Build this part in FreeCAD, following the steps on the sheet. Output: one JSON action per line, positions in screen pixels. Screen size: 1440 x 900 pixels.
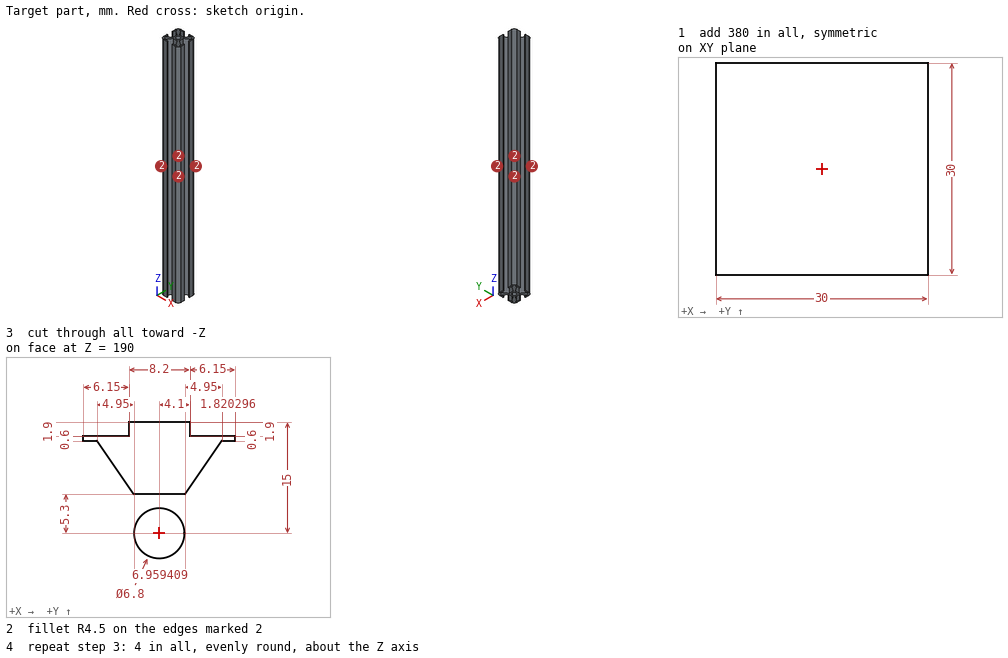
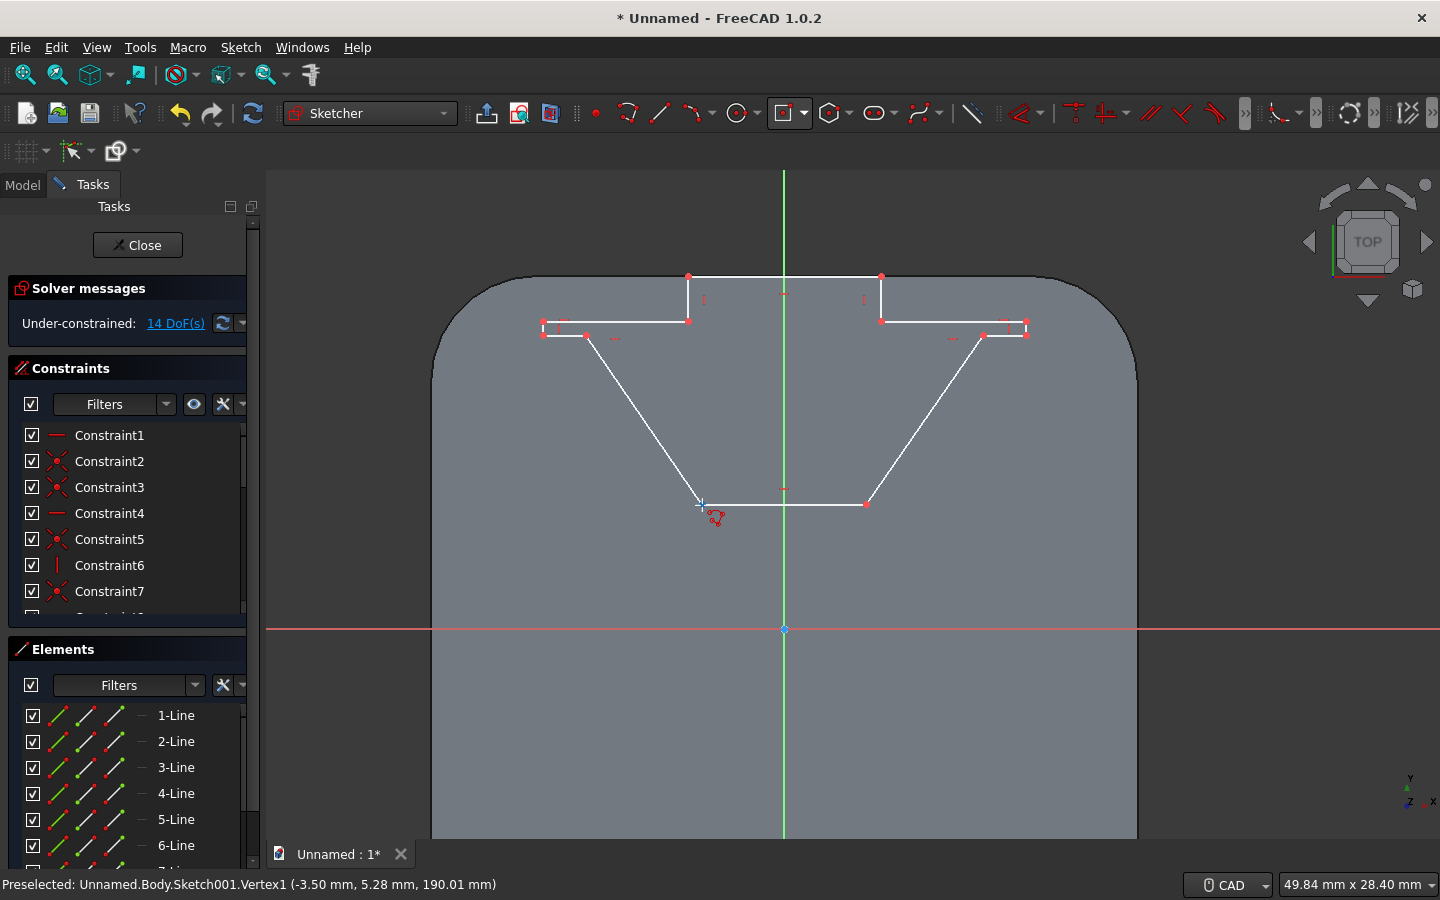
{"action": "left_click", "coordinate": [738, 114]}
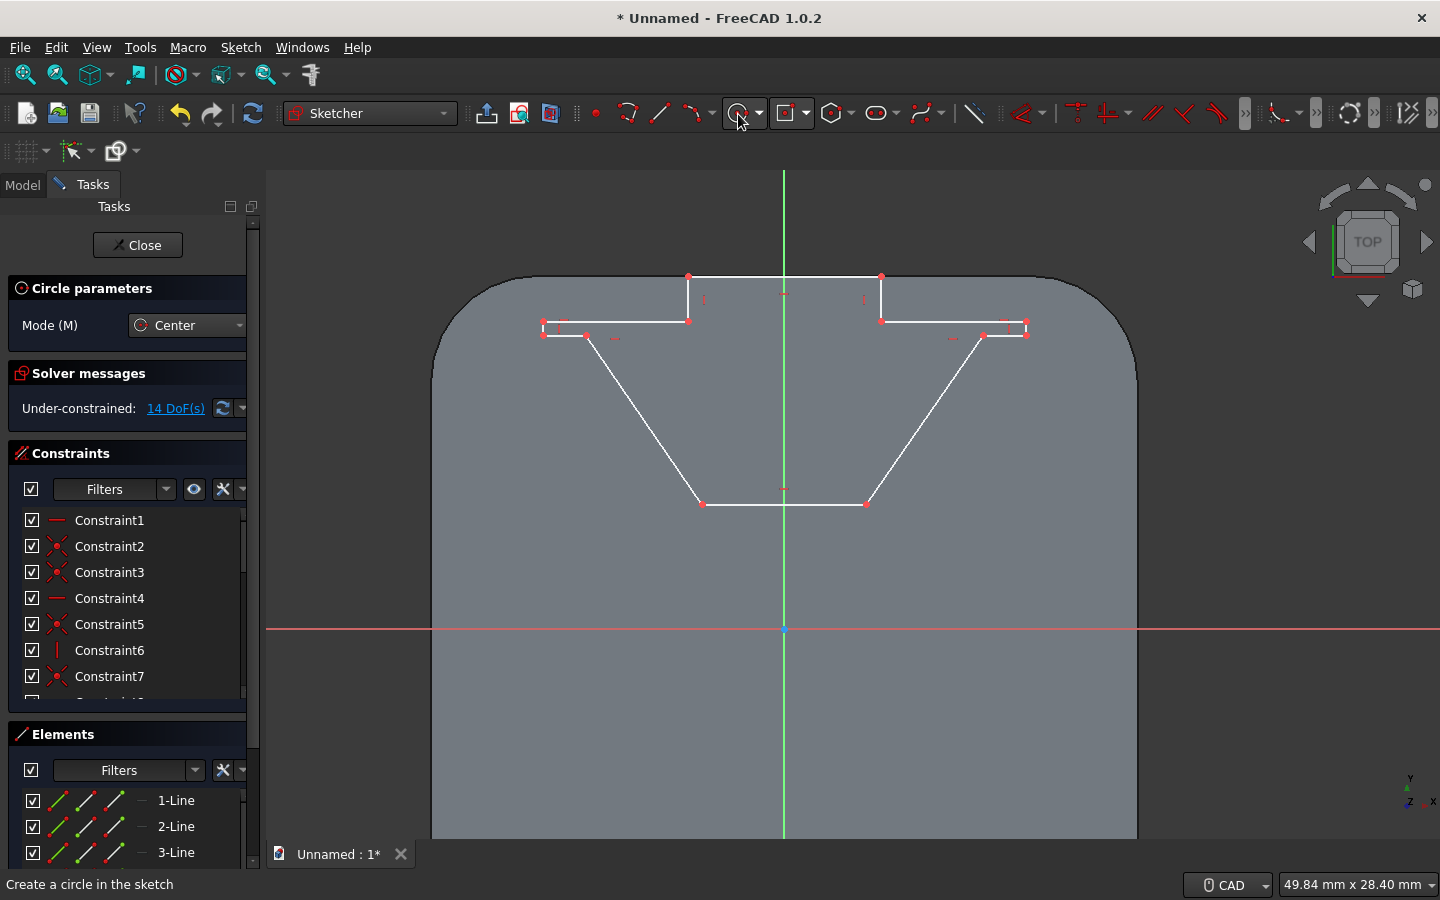
{"action": "left_click", "coordinate": [784, 629]}
{"action": "left_click", "coordinate": [841, 573]}
{"action": "key", "text": "Escape"}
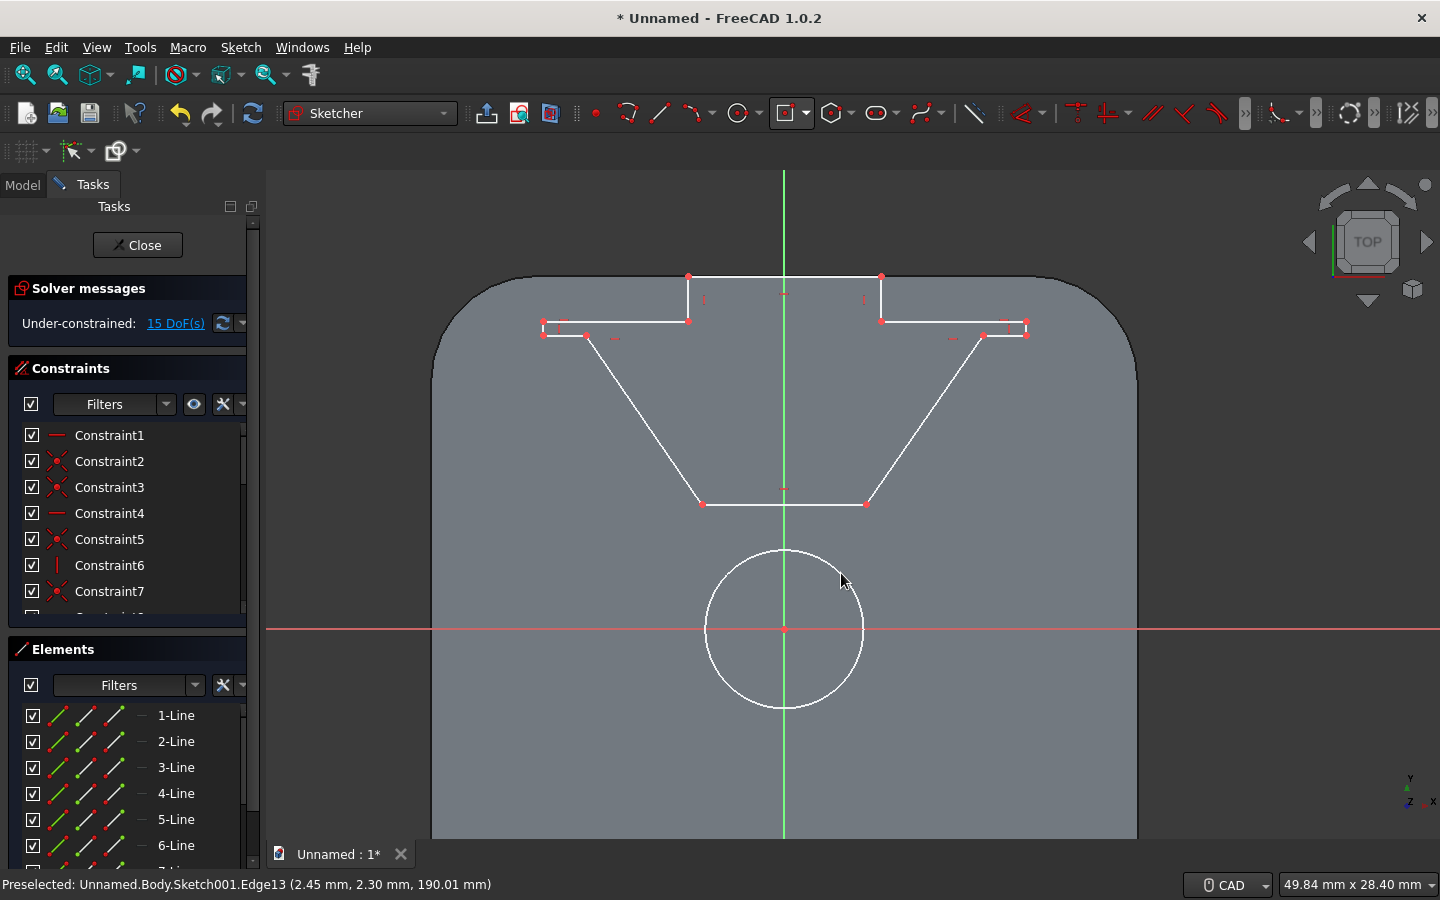
{"action": "left_click", "coordinate": [1022, 114]}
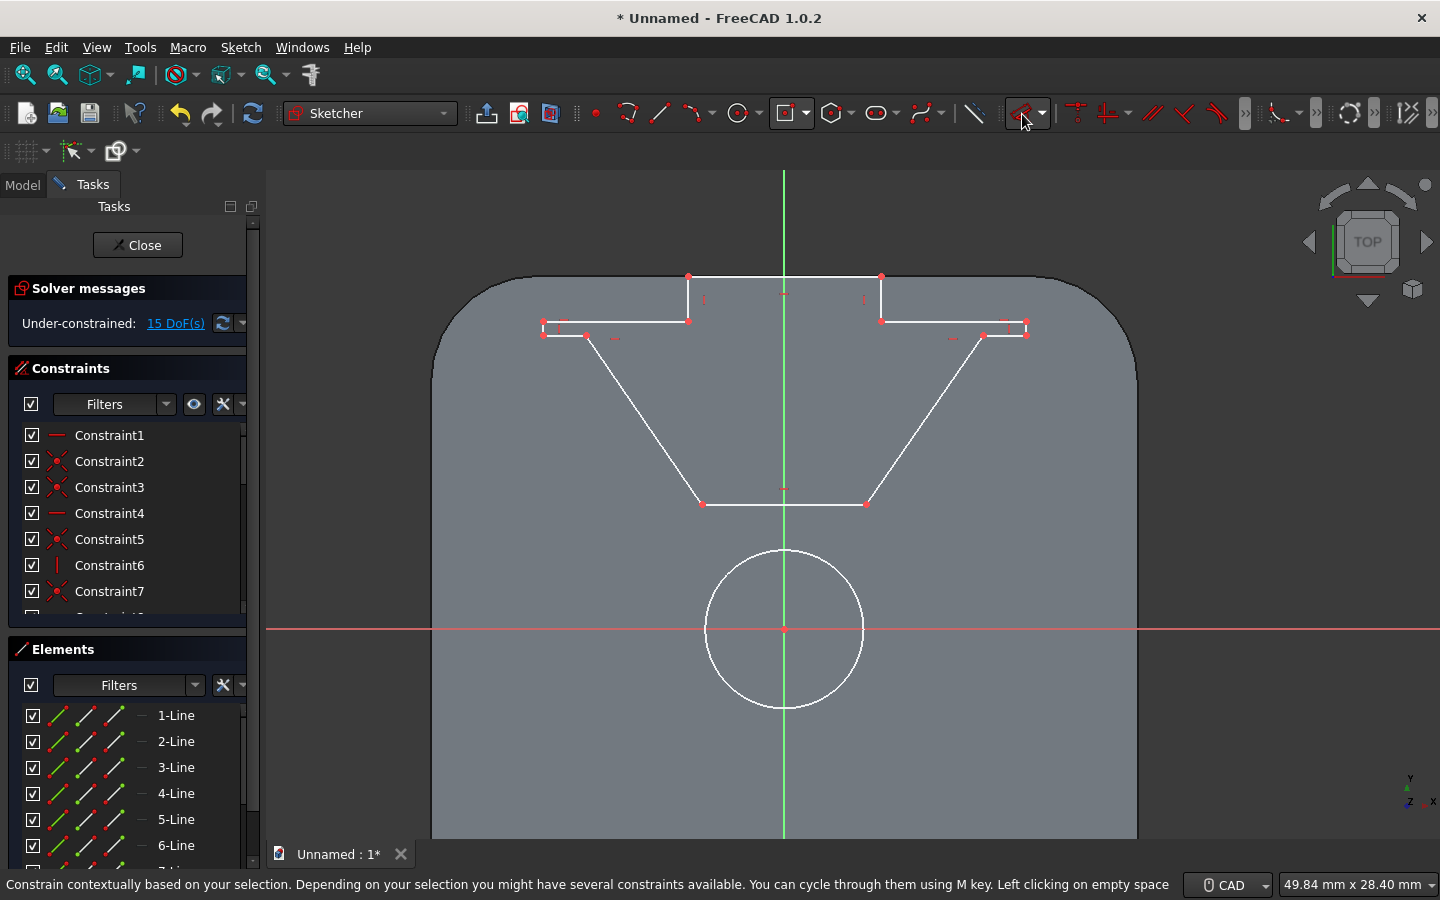
{"action": "left_click", "coordinate": [840, 573]}
{"action": "left_click", "coordinate": [862, 550]}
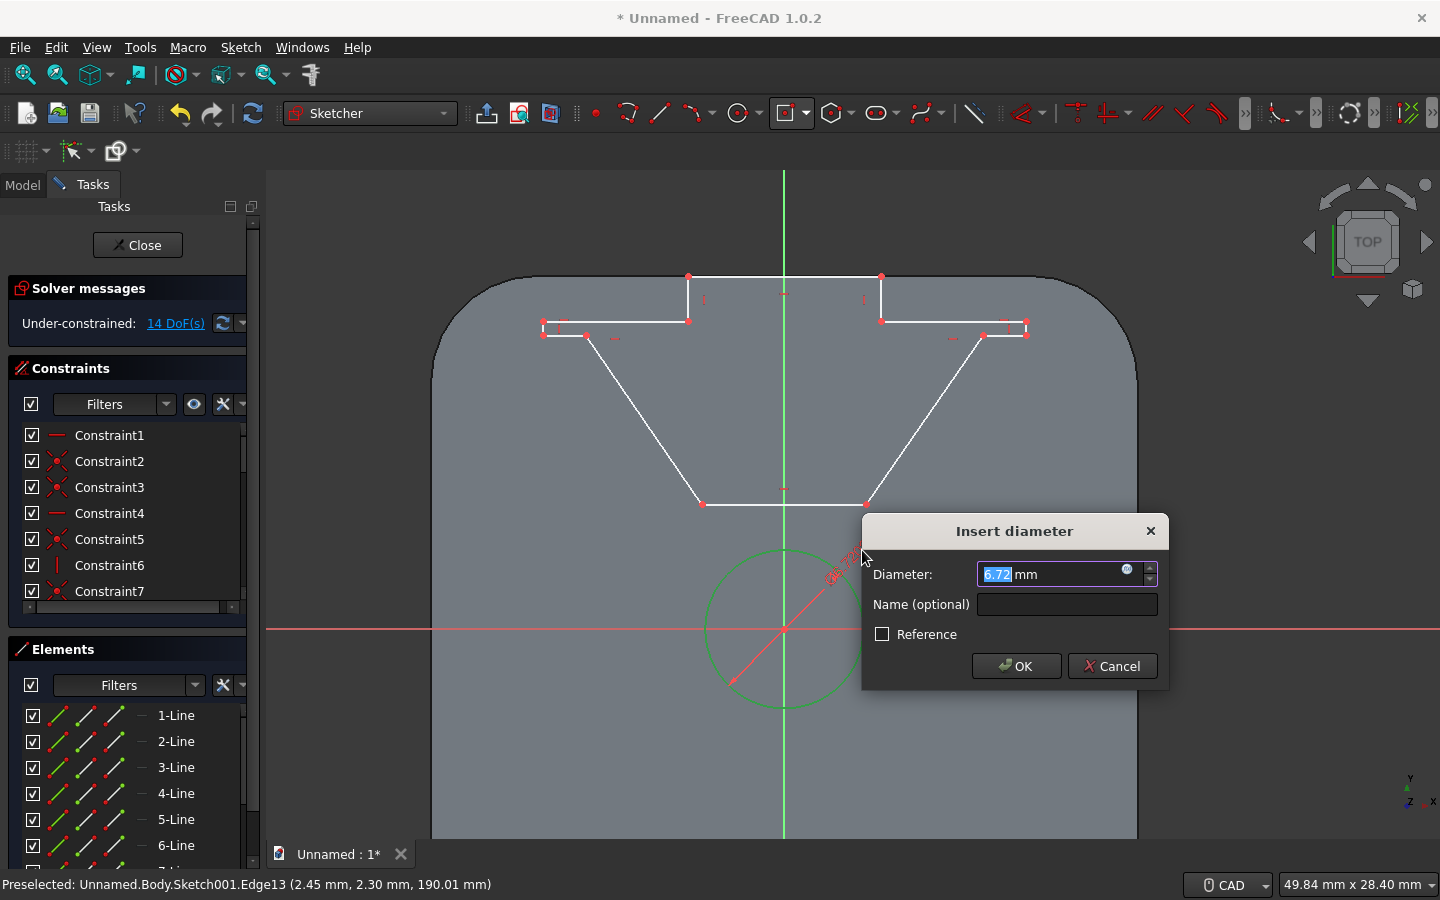
{"action": "type", "text": "6.8"}
{"action": "key", "text": "Return"}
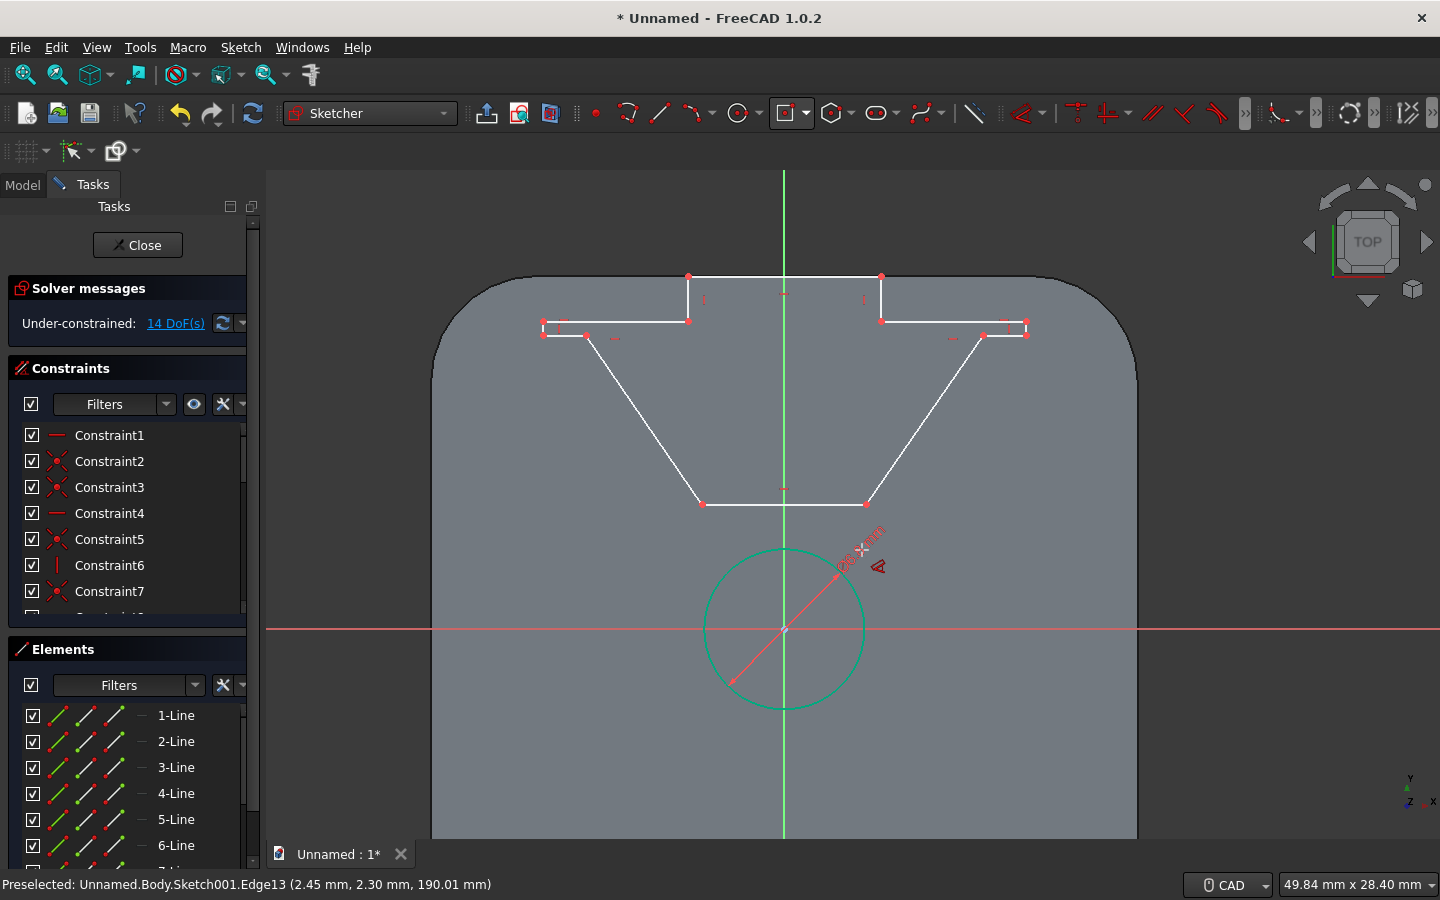
{"action": "scroll", "coordinate": [1026, 329], "scroll_direction": "up", "scroll_amount": 6}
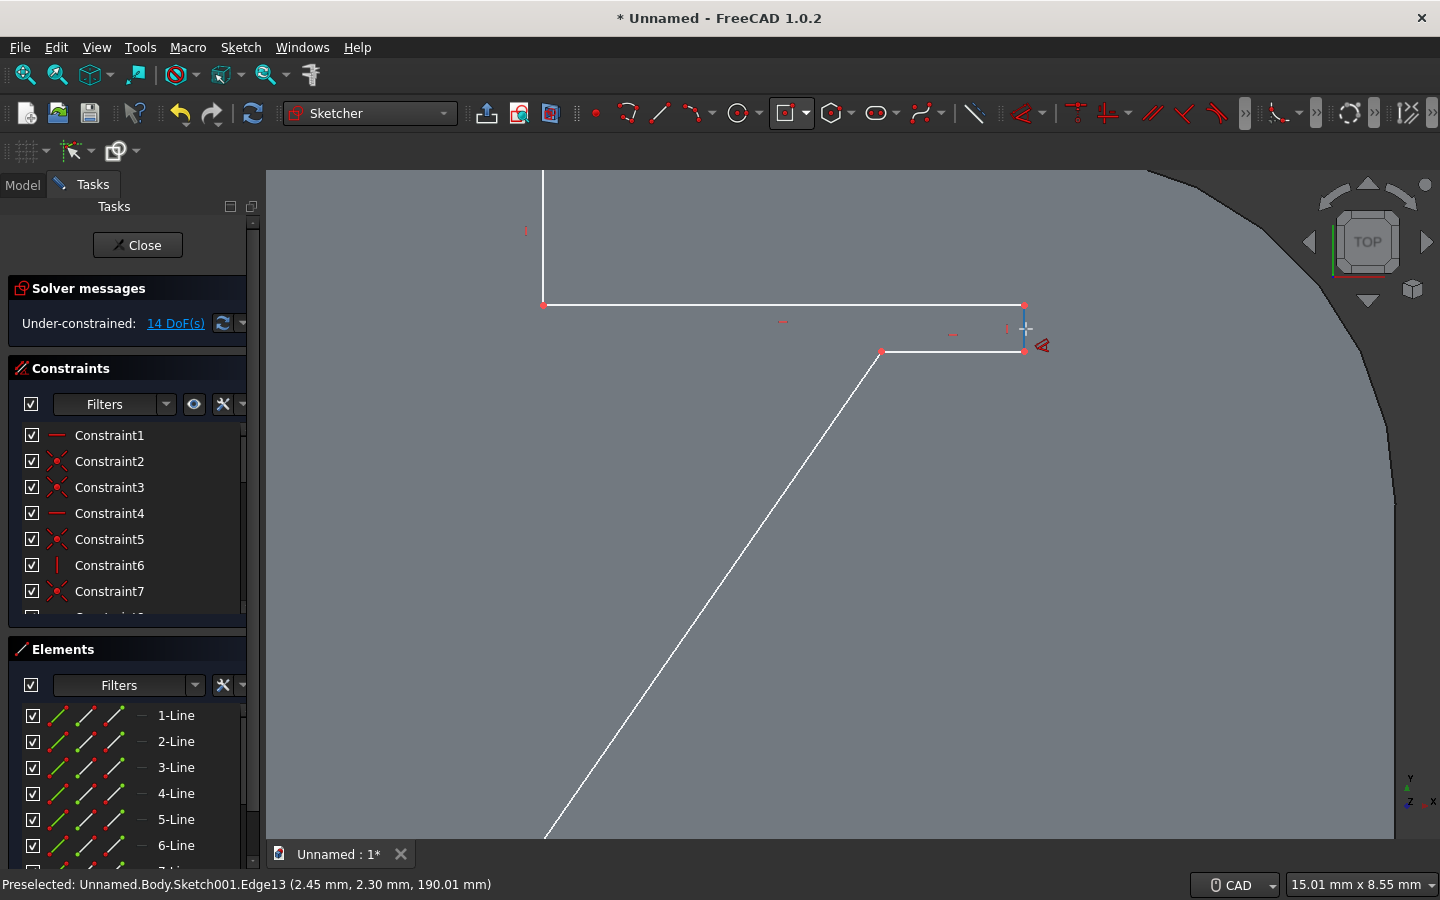
{"action": "left_click", "coordinate": [1024, 328]}
{"action": "left_click", "coordinate": [1058, 328]}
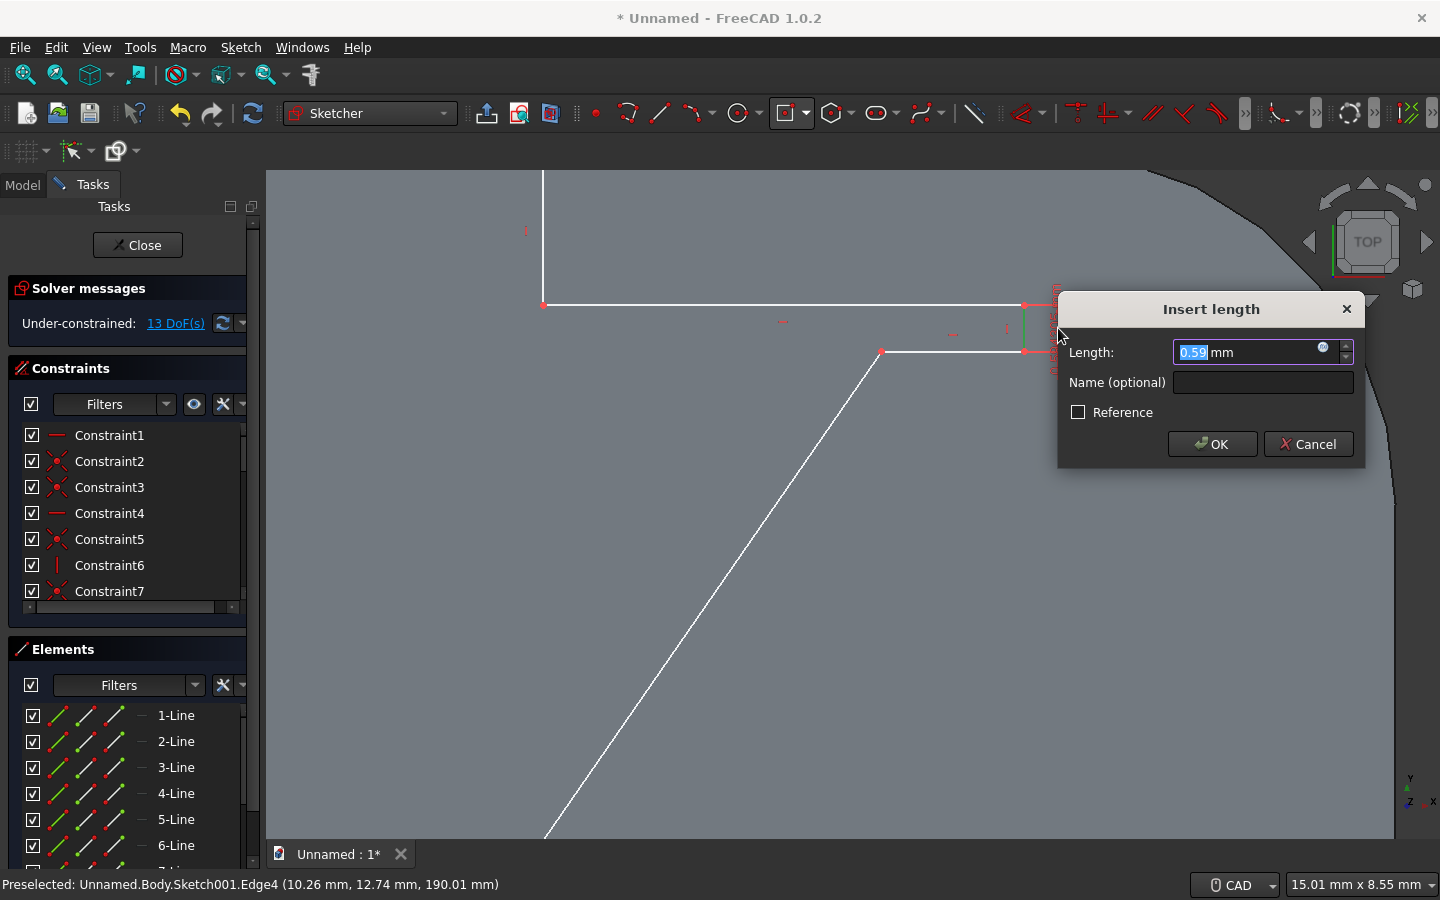
{"action": "type", "text": "0.6"}
{"action": "key", "text": "Return"}